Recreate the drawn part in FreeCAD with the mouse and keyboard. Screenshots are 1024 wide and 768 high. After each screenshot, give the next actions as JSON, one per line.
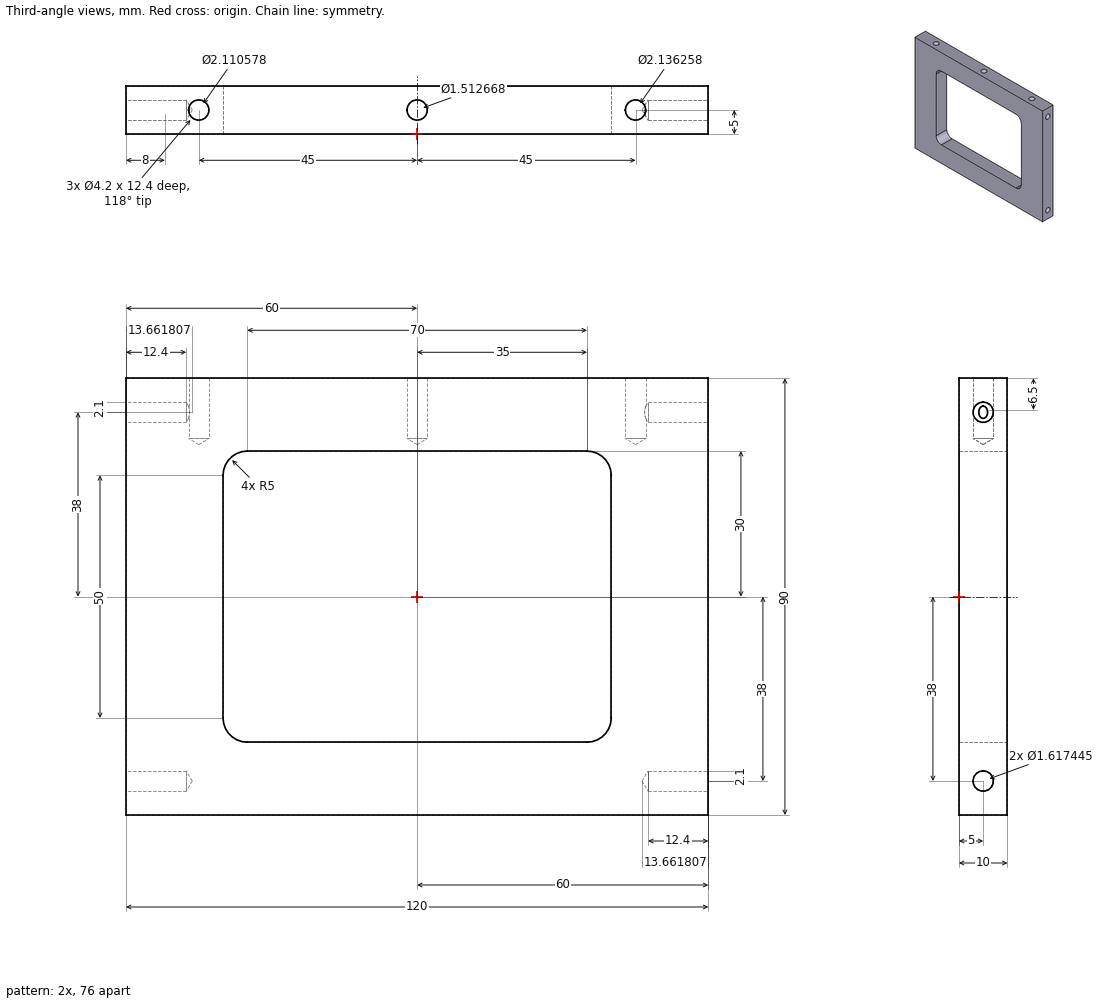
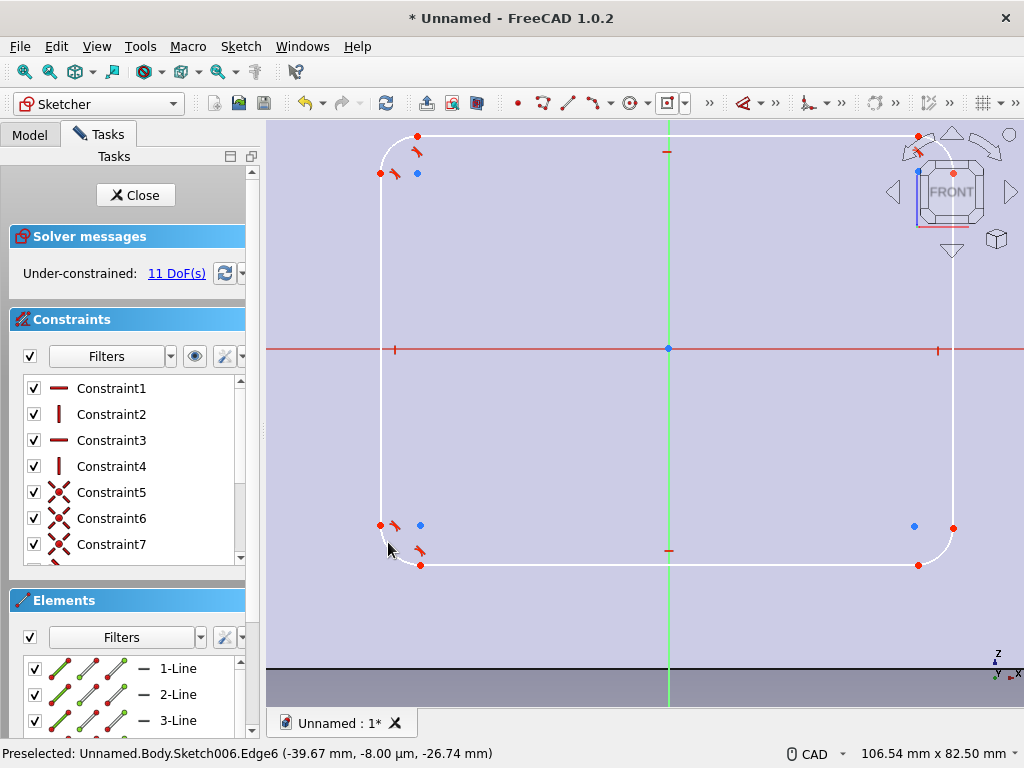
{"action": "left_click", "coordinate": [570, 565]}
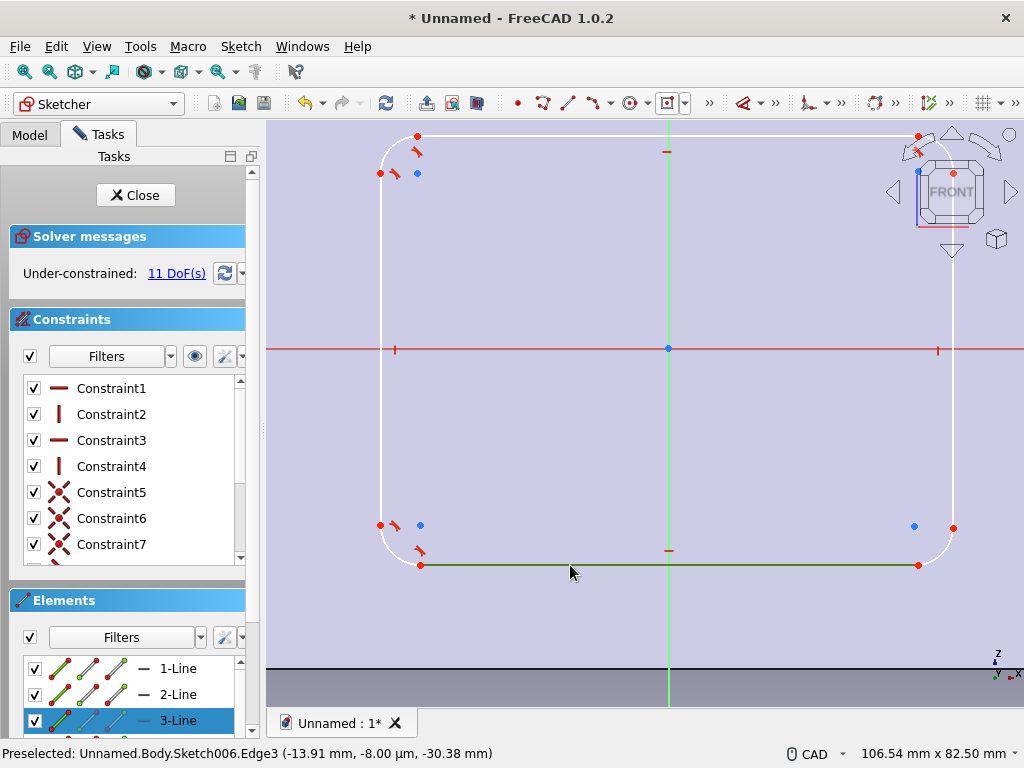
{"action": "scroll", "coordinate": [388, 545], "scroll_direction": "down", "scroll_amount": 2}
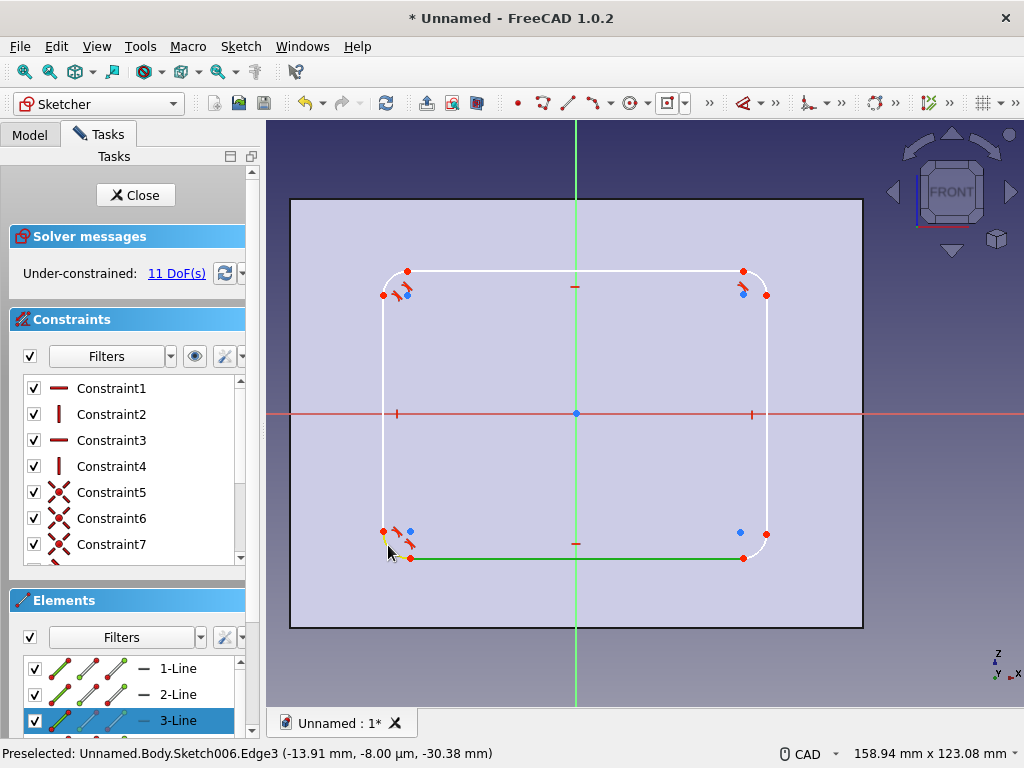
{"action": "scroll", "coordinate": [754, 555], "scroll_direction": "up", "scroll_amount": 2}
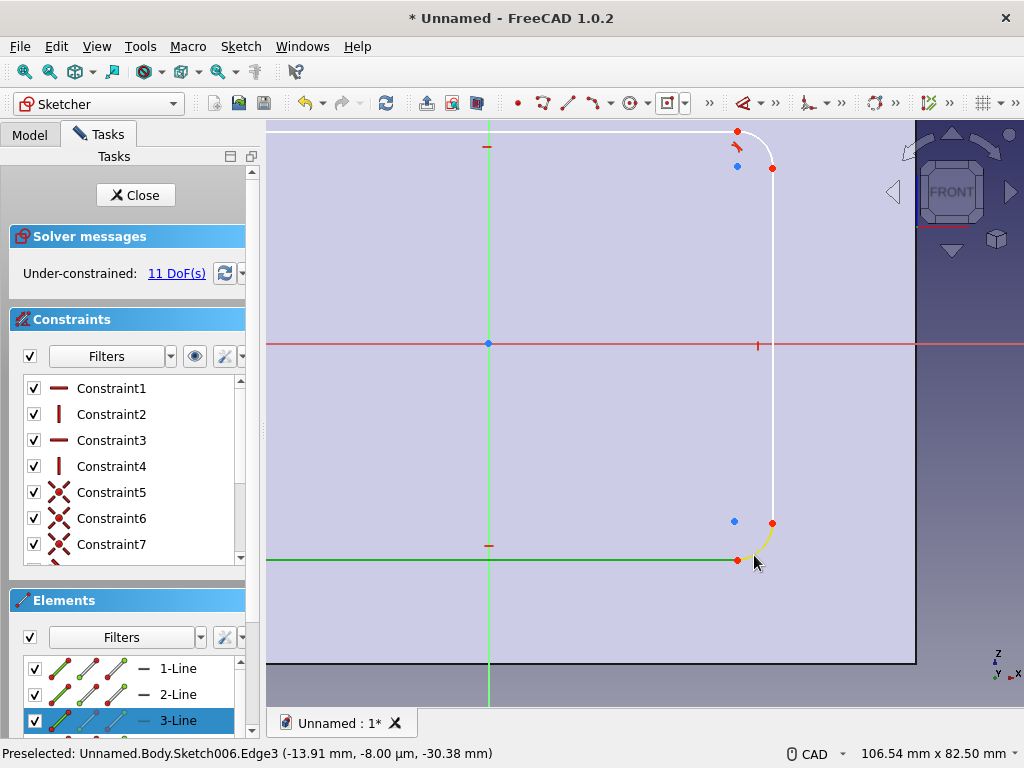
{"action": "left_click", "coordinate": [754, 555]}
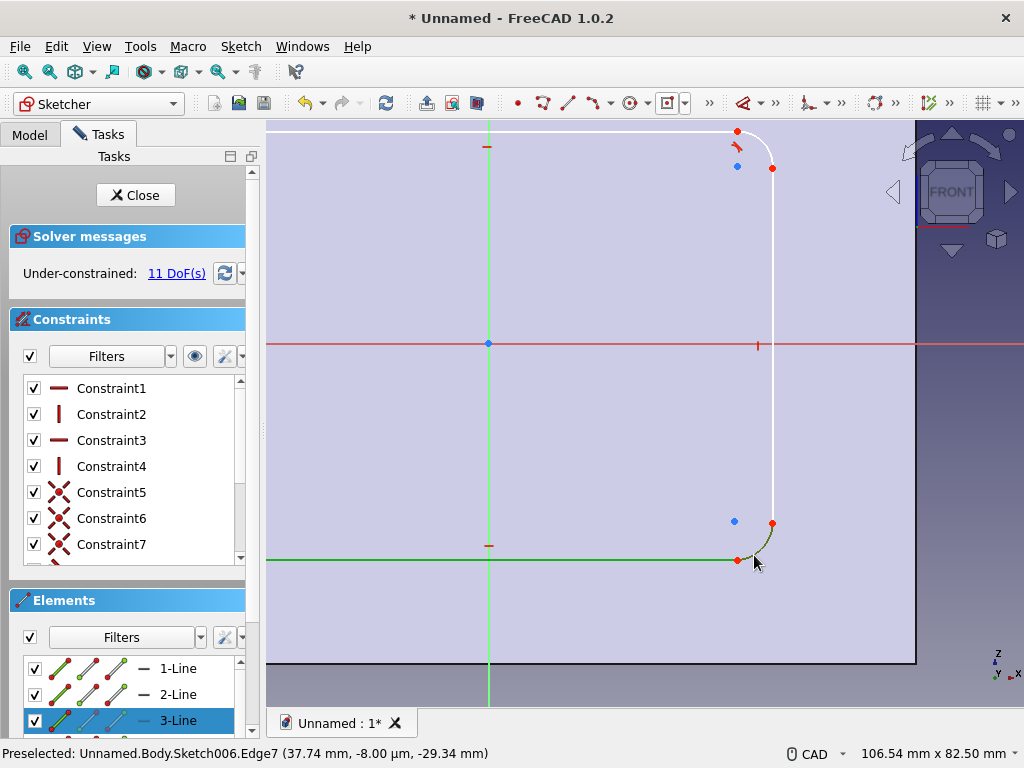
{"action": "key", "text": "t"}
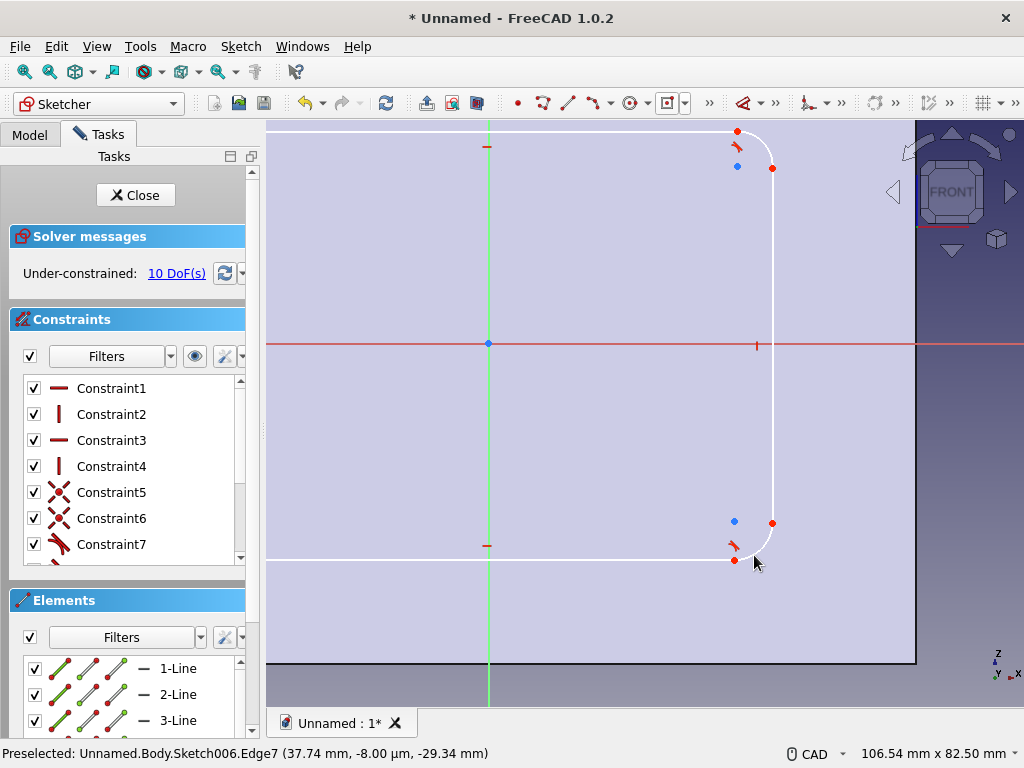
{"action": "left_click", "coordinate": [773, 417]}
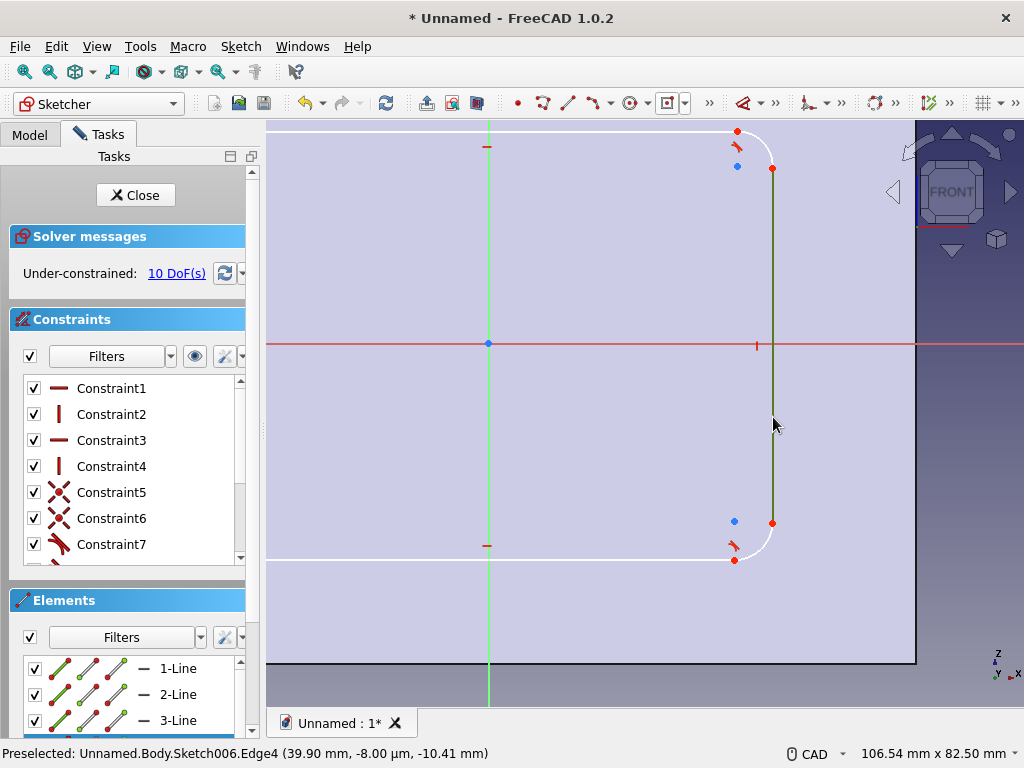
{"action": "left_click", "coordinate": [751, 556]}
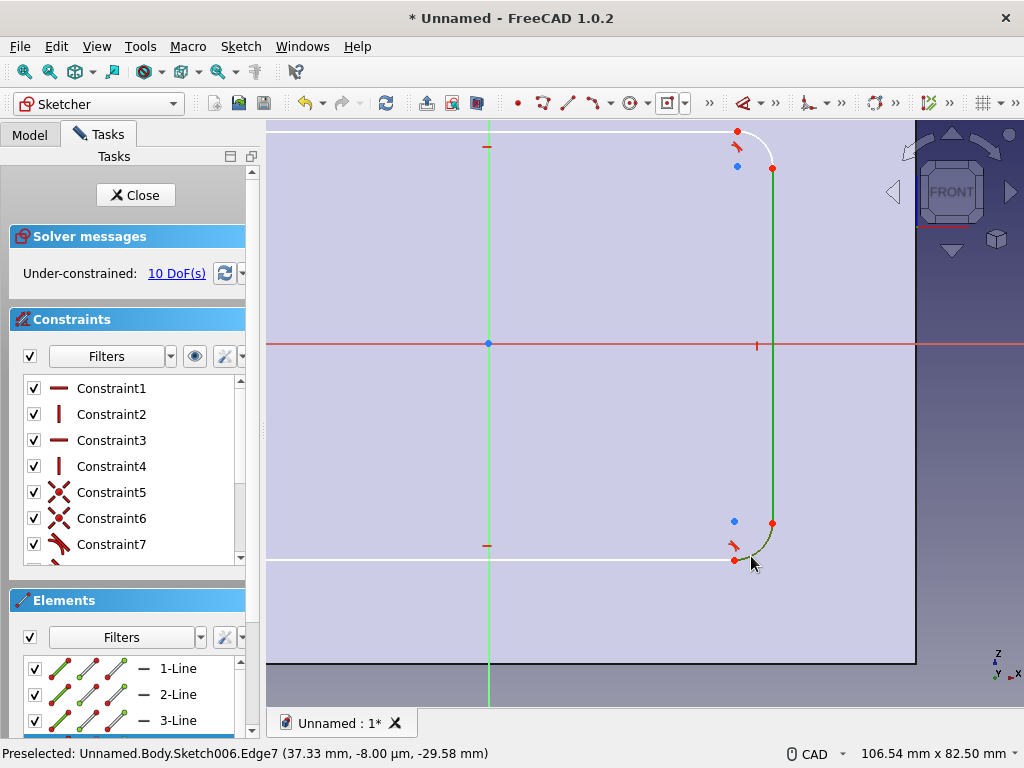
{"action": "key", "text": "t"}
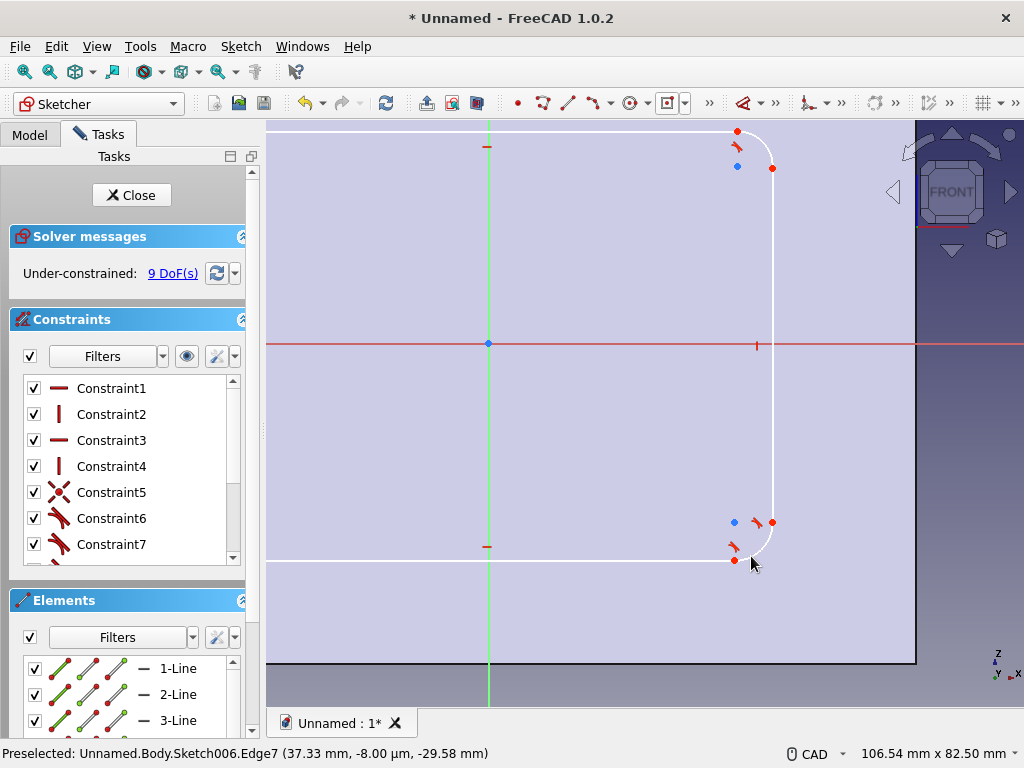
{"action": "left_click", "coordinate": [773, 416]}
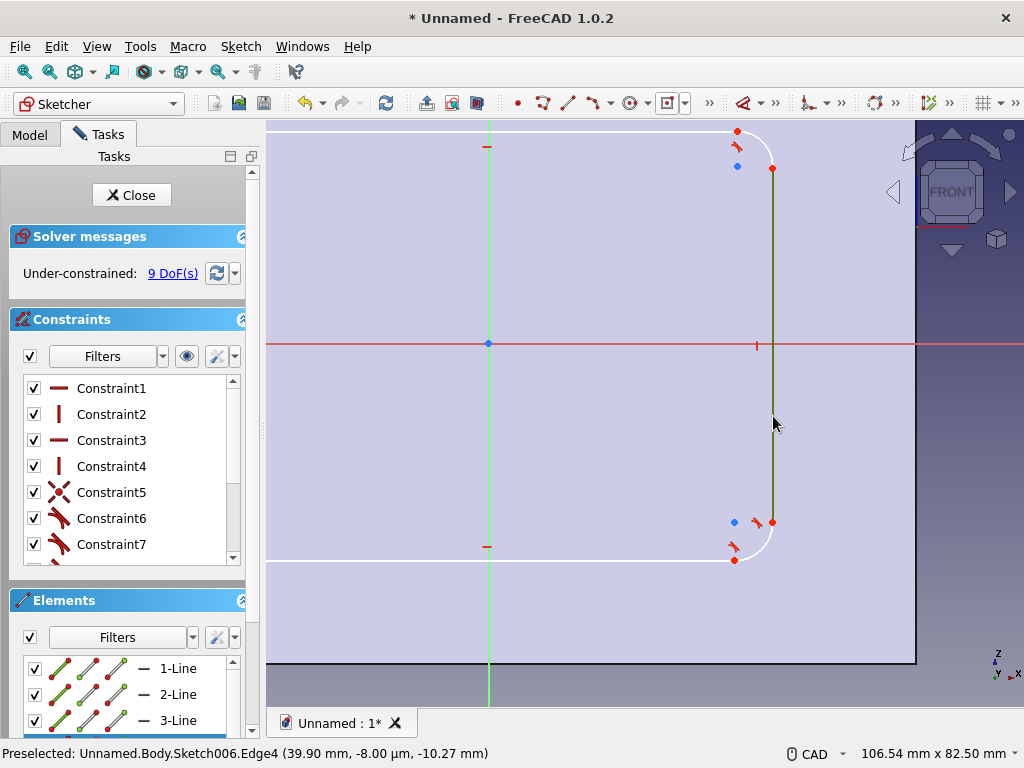
{"action": "left_click", "coordinate": [769, 152]}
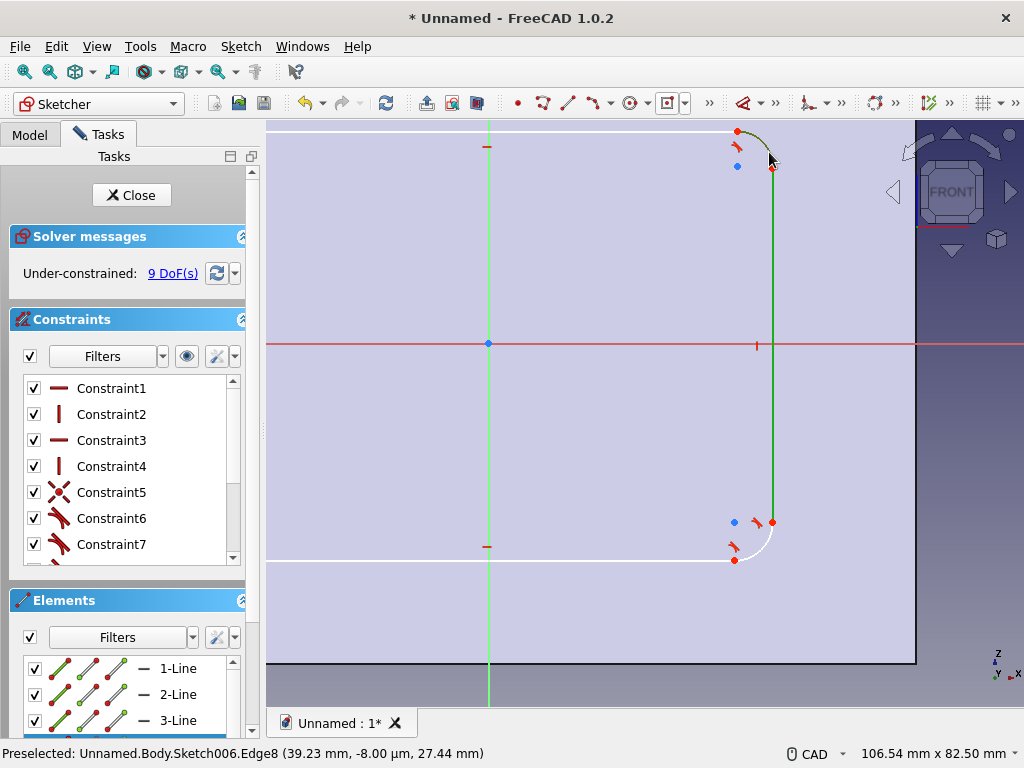
{"action": "key", "text": "t"}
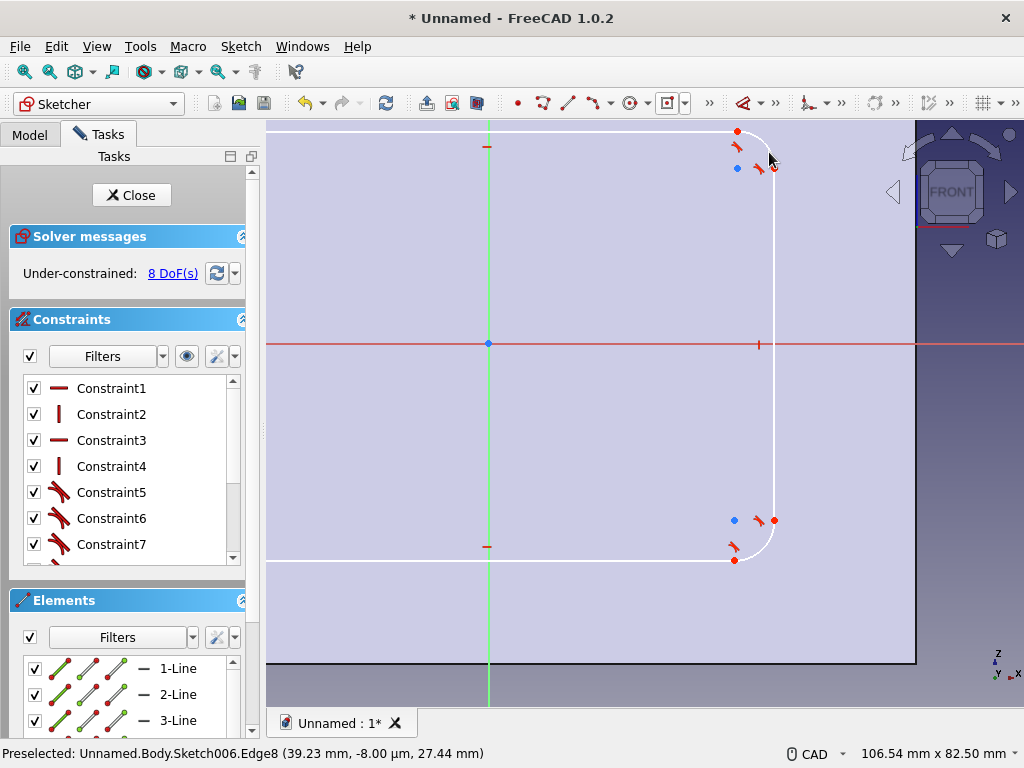
{"action": "scroll", "coordinate": [755, 555], "scroll_direction": "down", "scroll_amount": 2}